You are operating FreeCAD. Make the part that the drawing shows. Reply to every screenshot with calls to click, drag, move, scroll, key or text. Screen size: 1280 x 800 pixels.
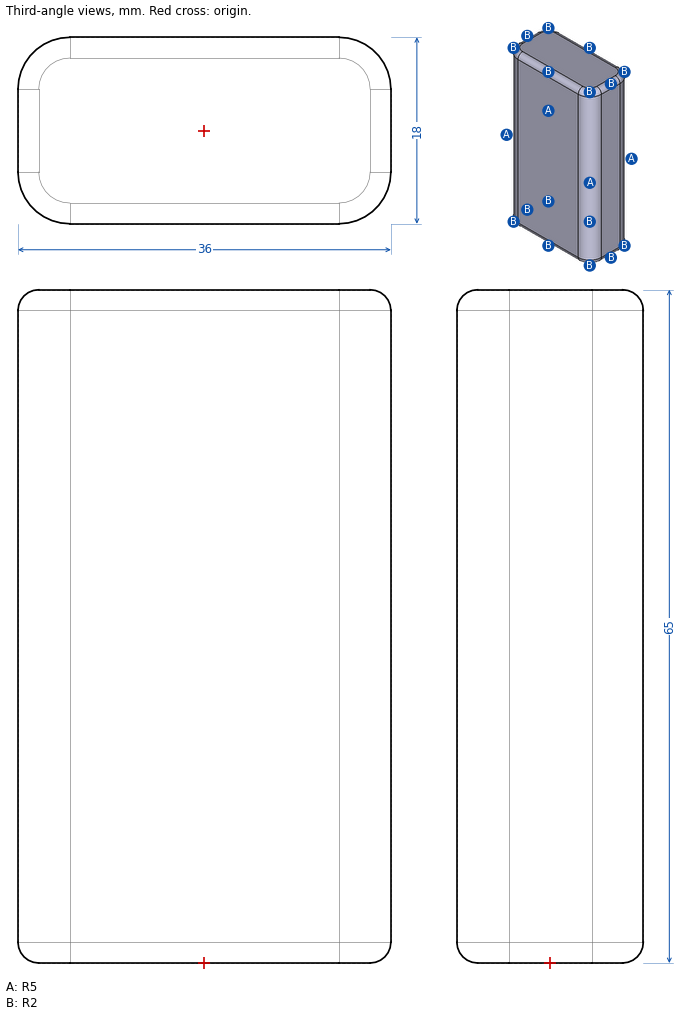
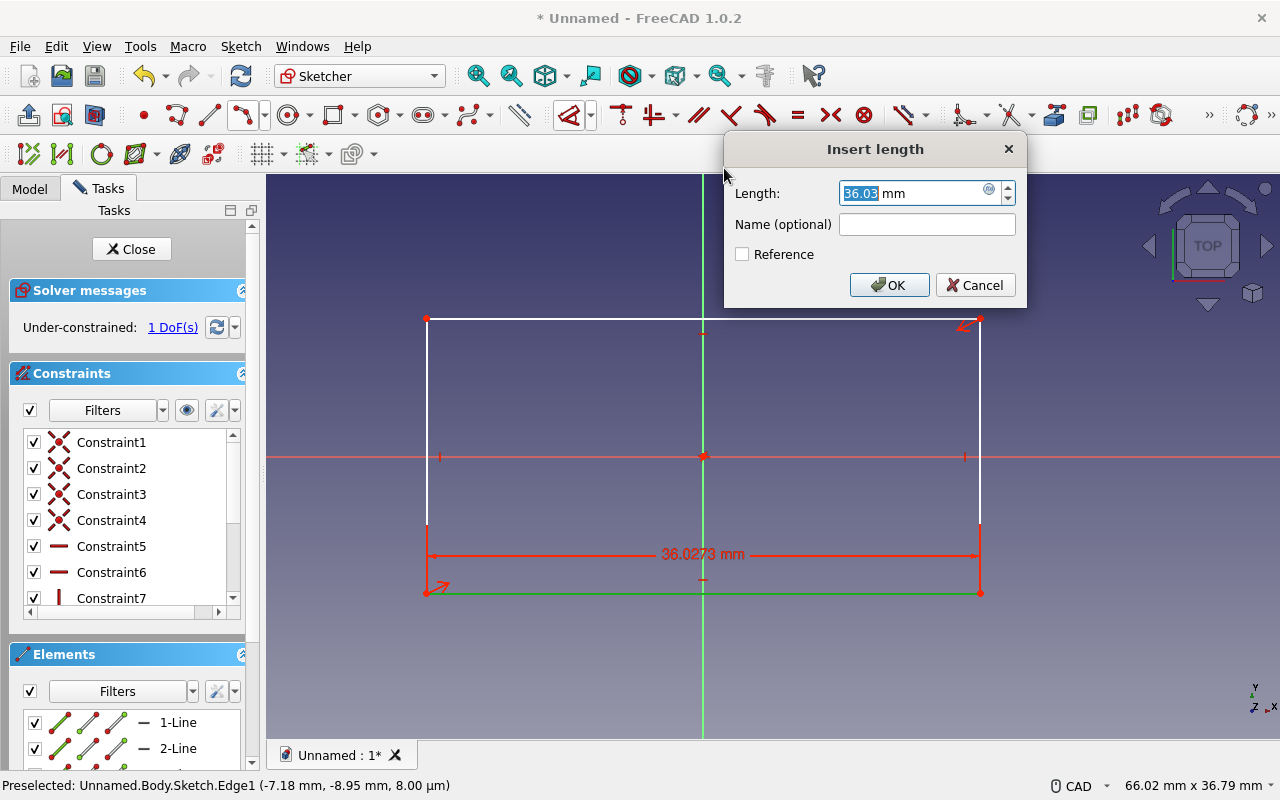
text(36)
key(Return)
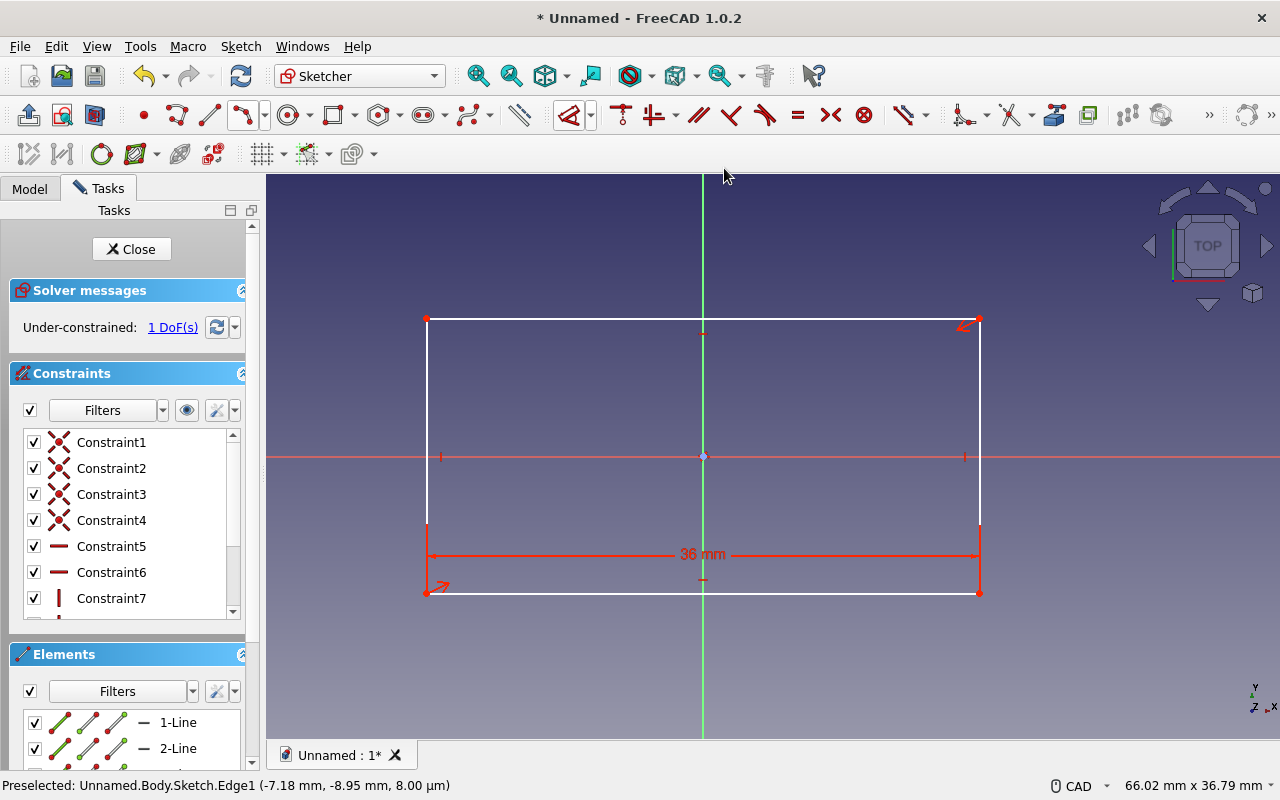
click(980, 512)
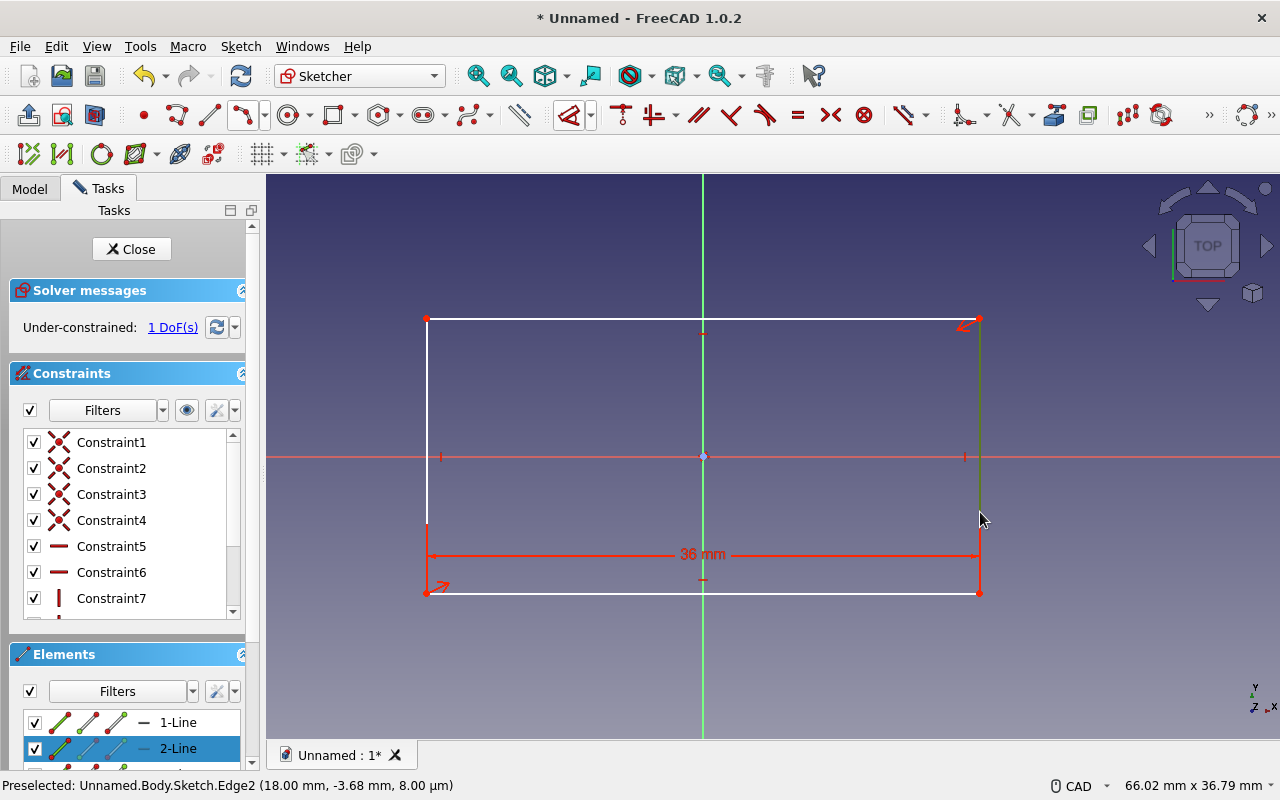
click(590, 116)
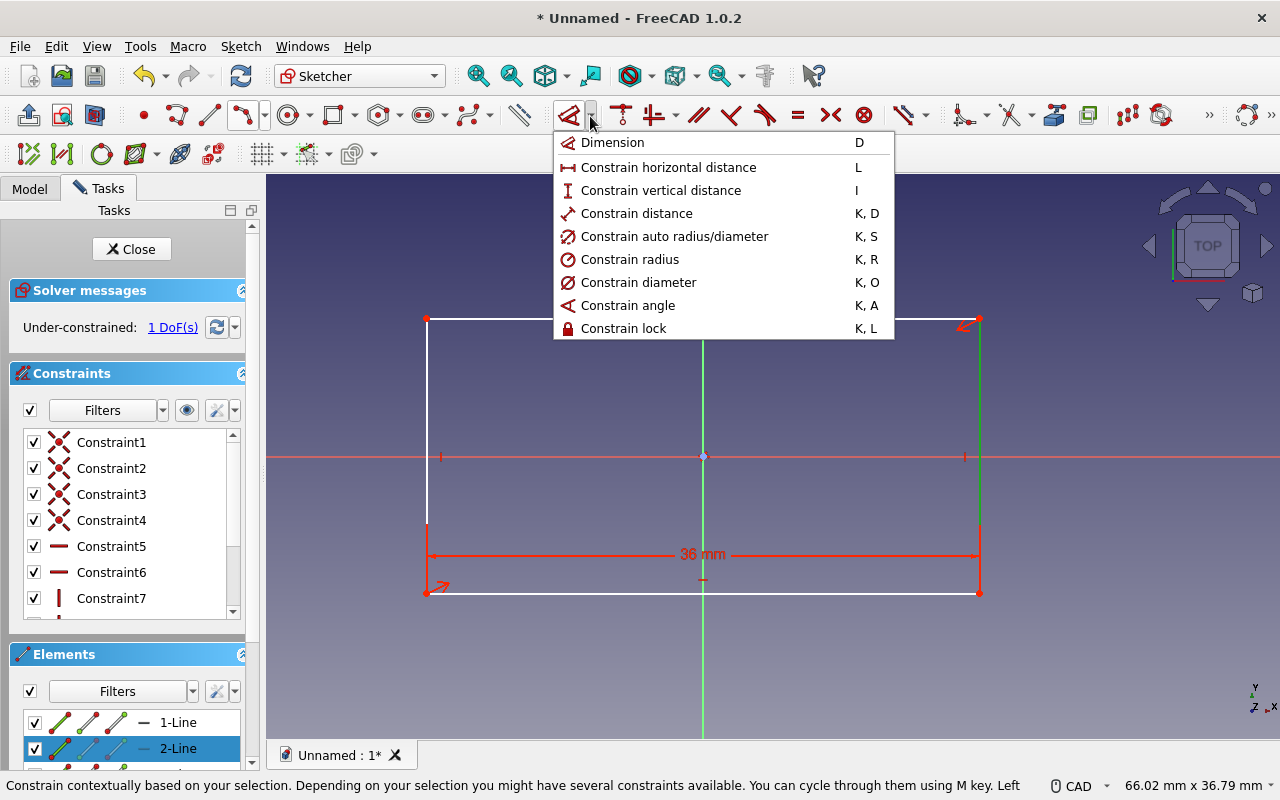
click(724, 190)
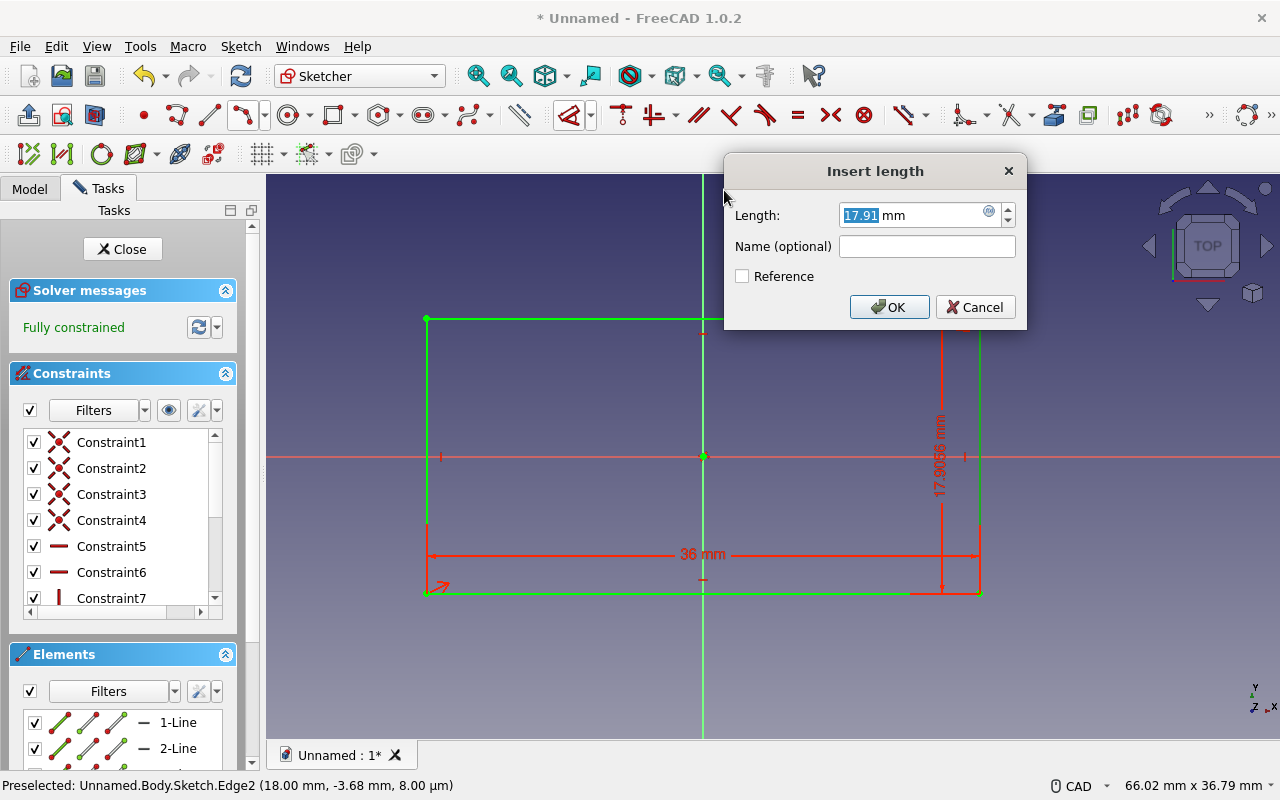
text(18)
key(Return)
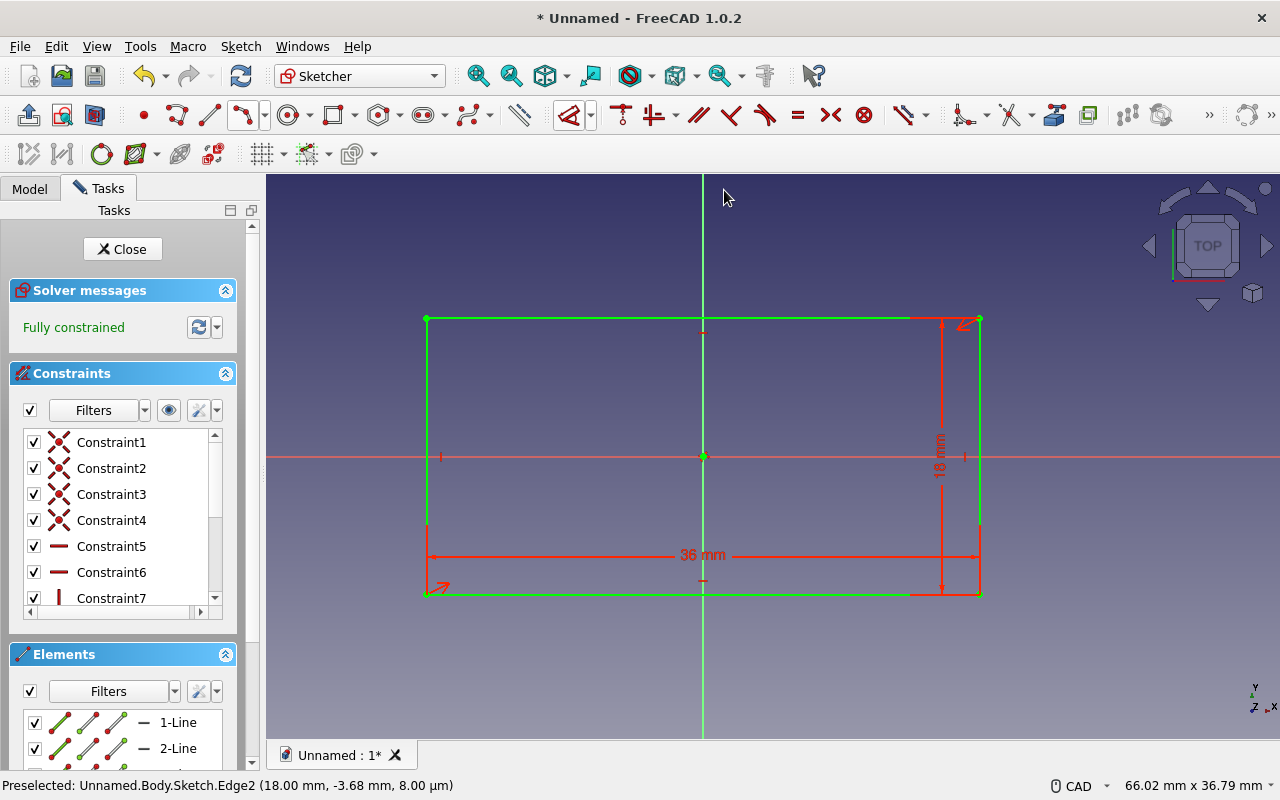
click(123, 249)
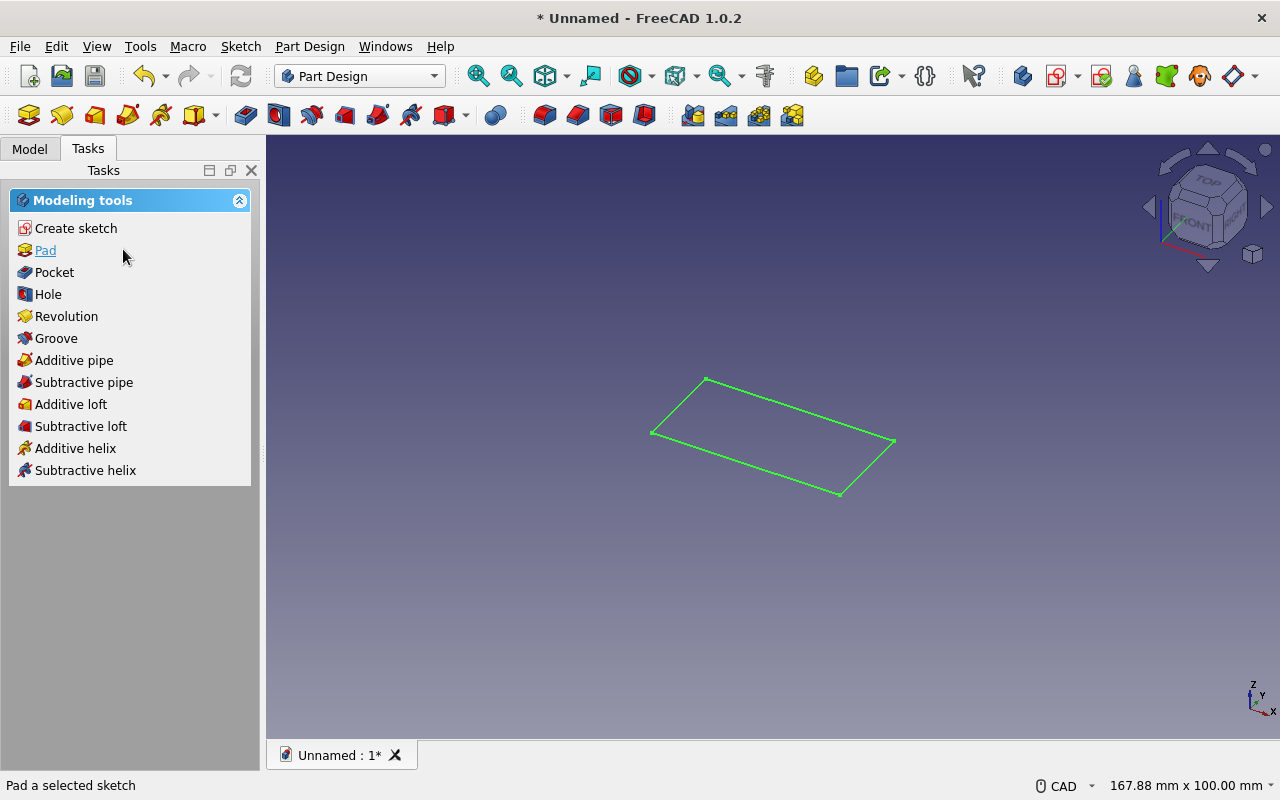
click(29, 116)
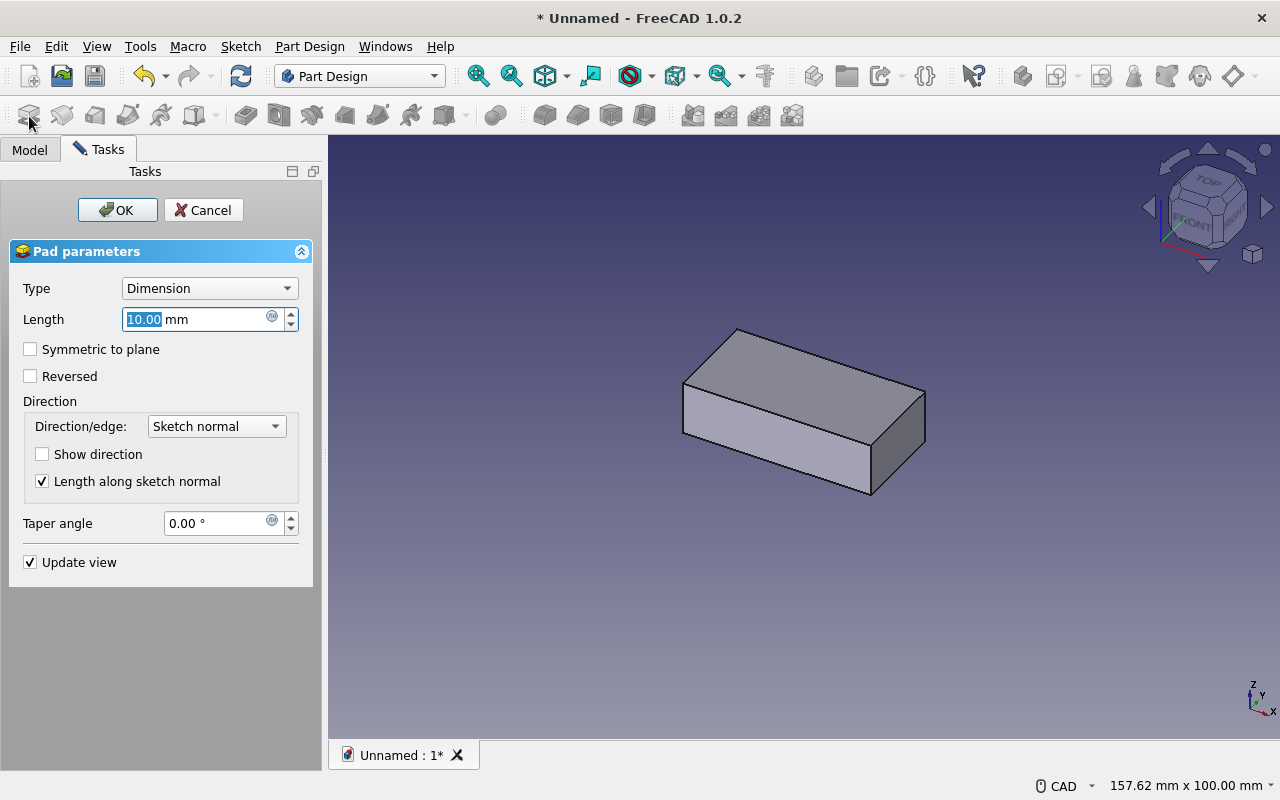
text(65)
key(Tab)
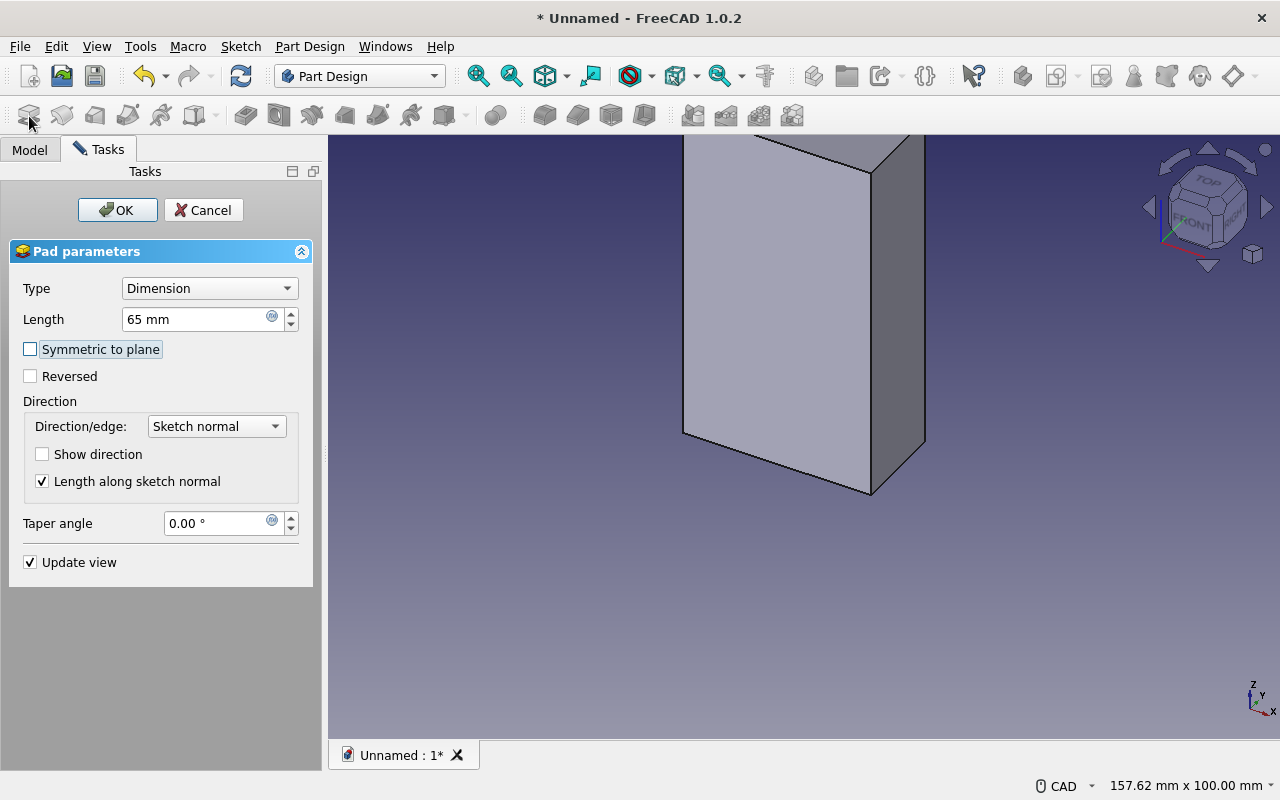
click(118, 210)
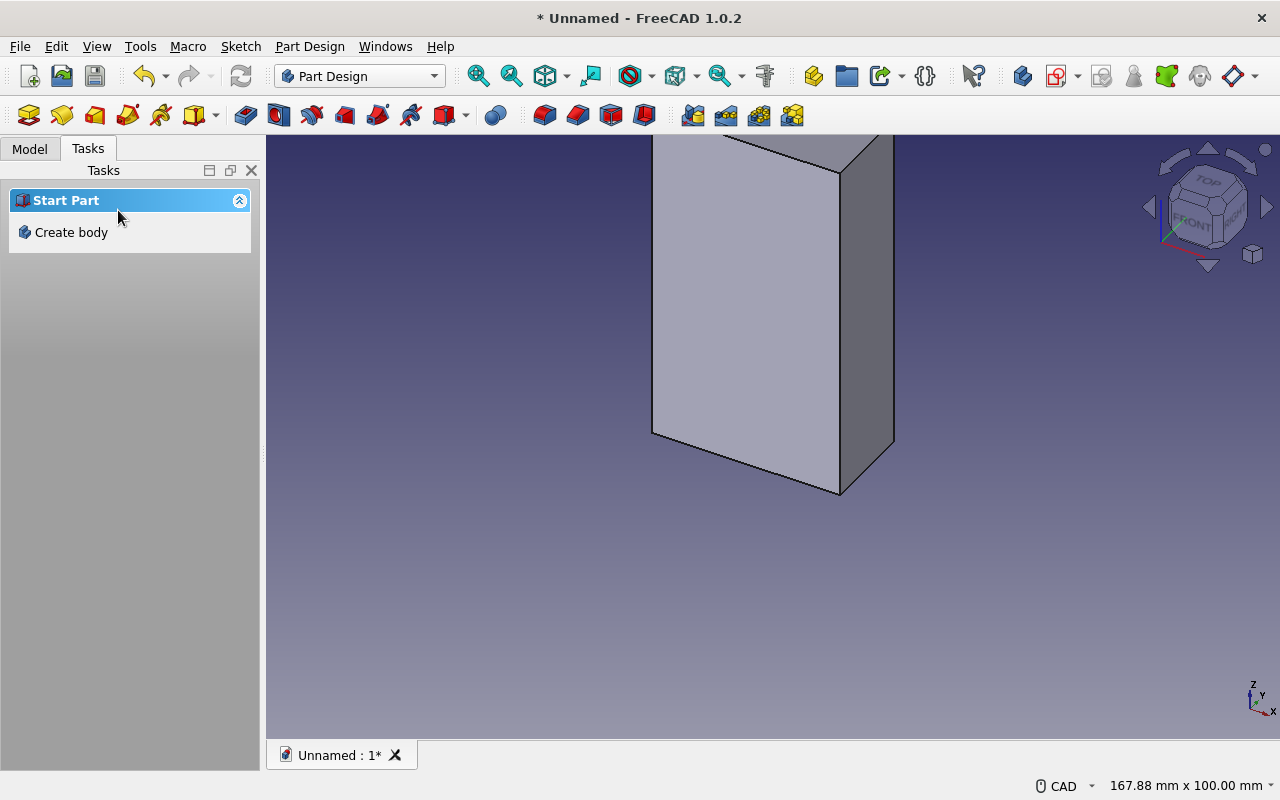
click(479, 76)